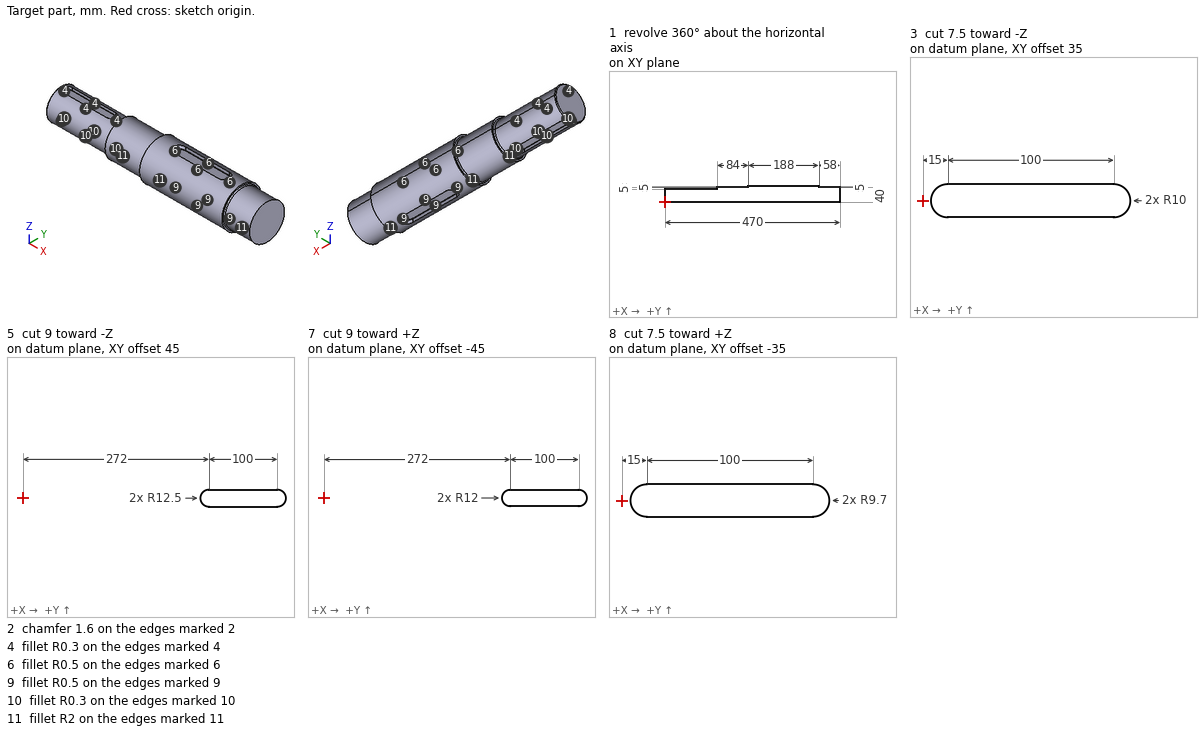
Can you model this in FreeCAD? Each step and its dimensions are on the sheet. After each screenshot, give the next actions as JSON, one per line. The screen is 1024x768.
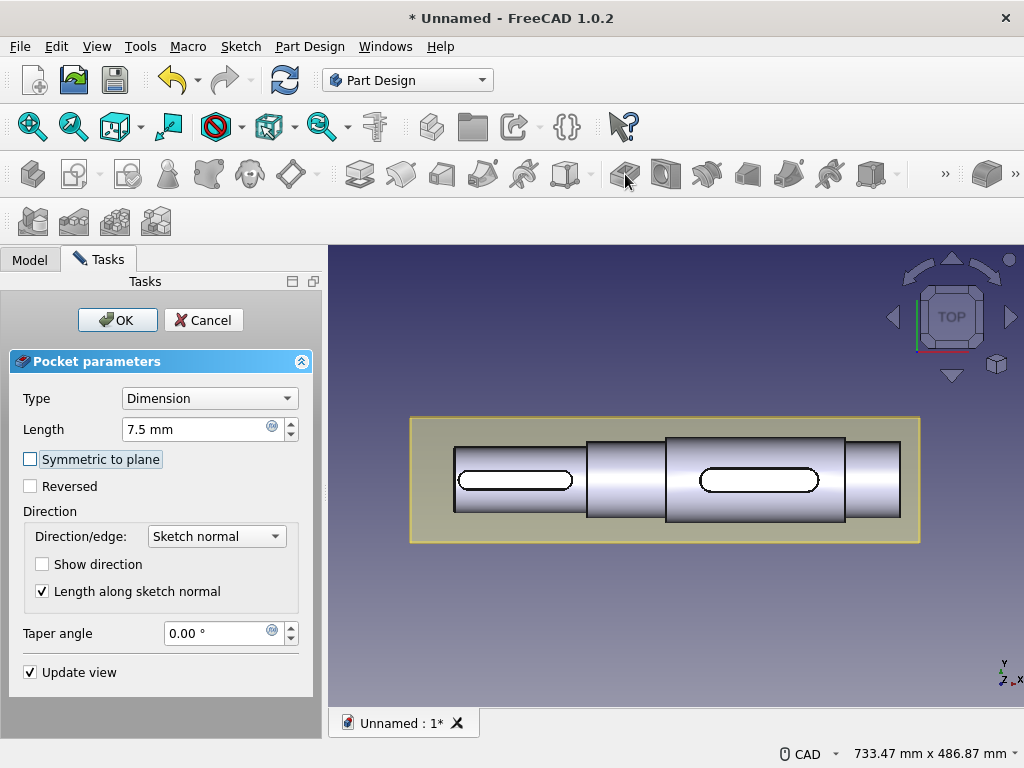
{"action": "left_click", "coordinate": [31, 486]}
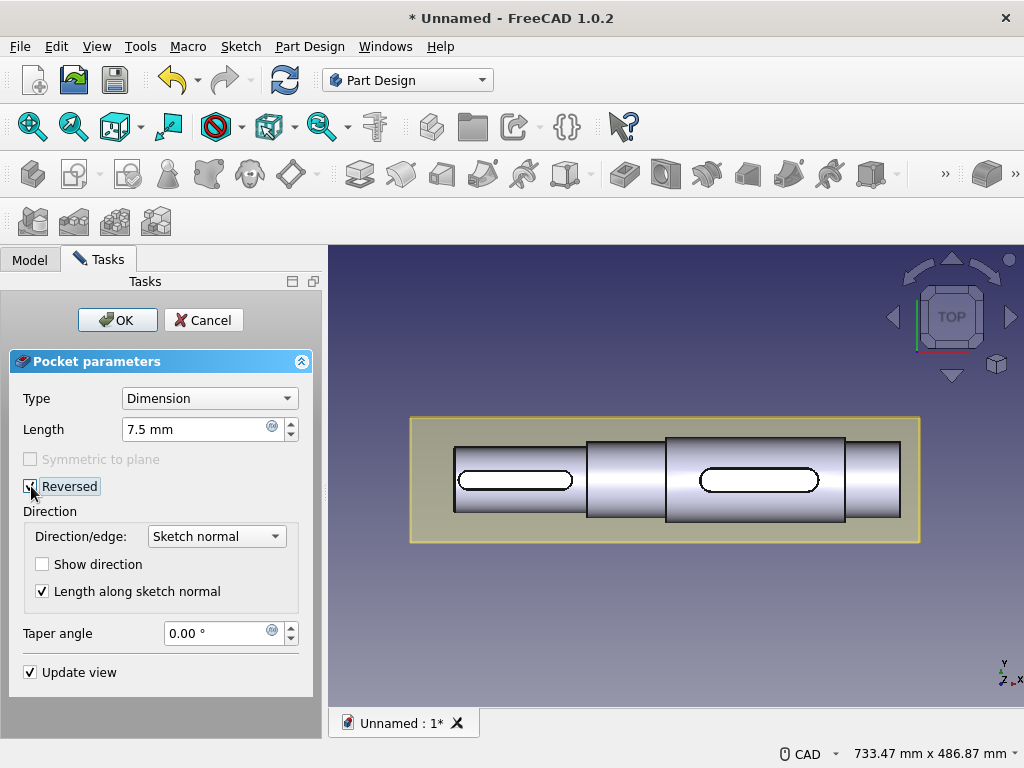
{"action": "left_click", "coordinate": [118, 320]}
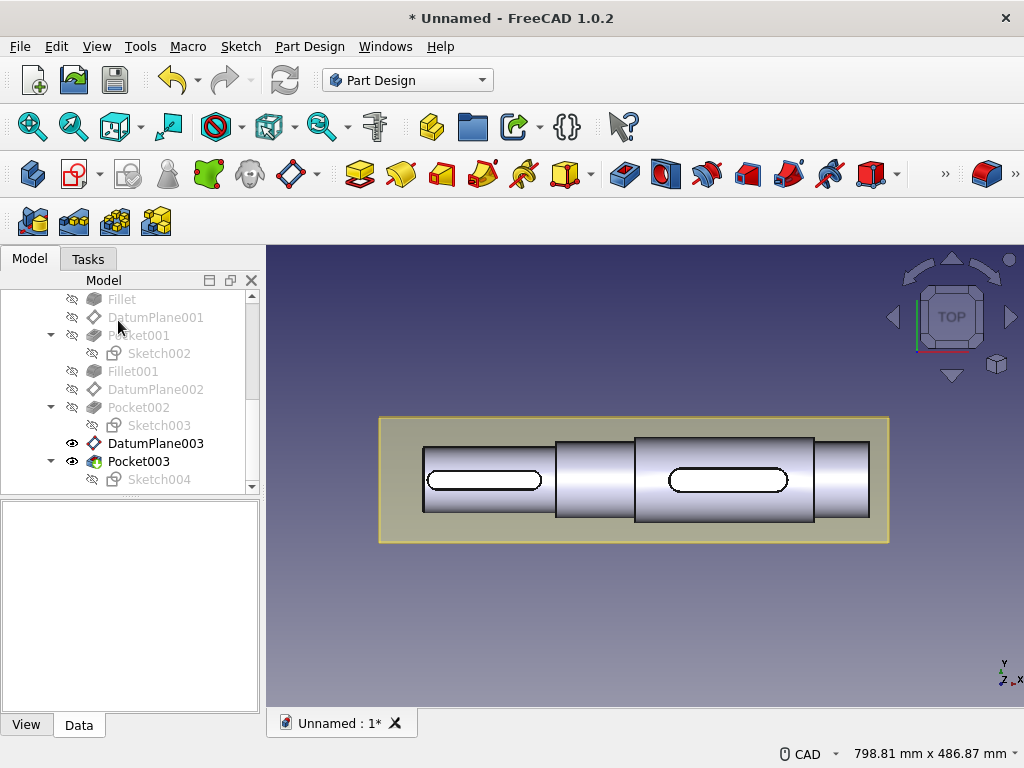
{"action": "left_click", "coordinate": [117, 443]}
{"action": "key", "text": "space"}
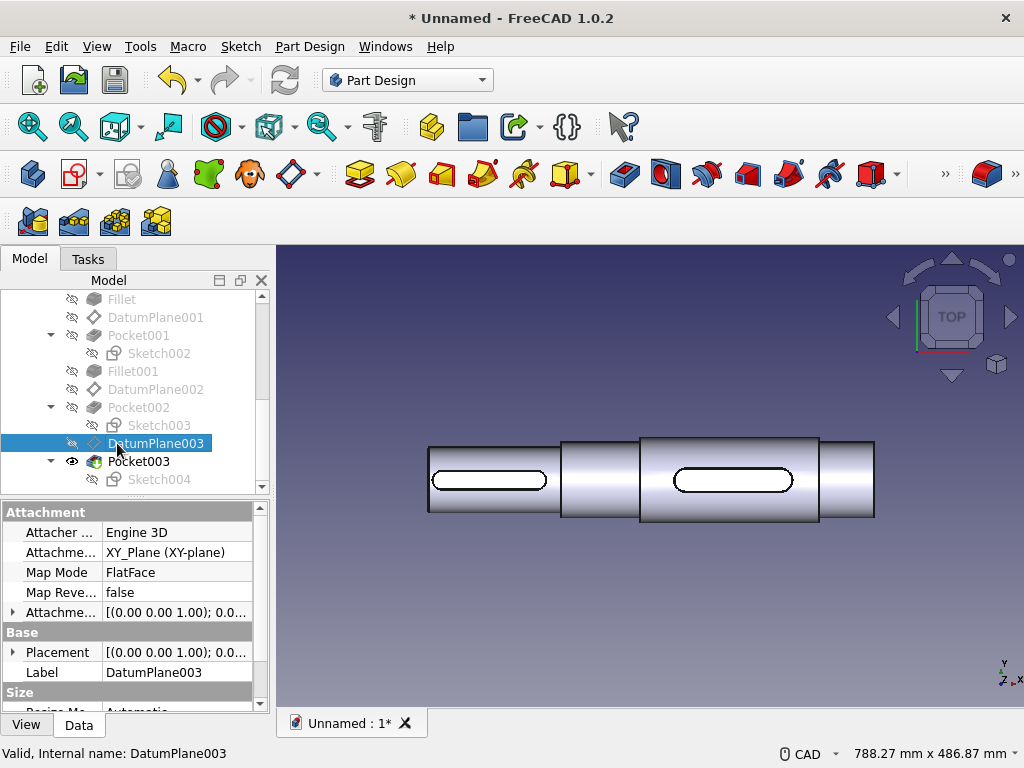
{"action": "key", "text": "0"}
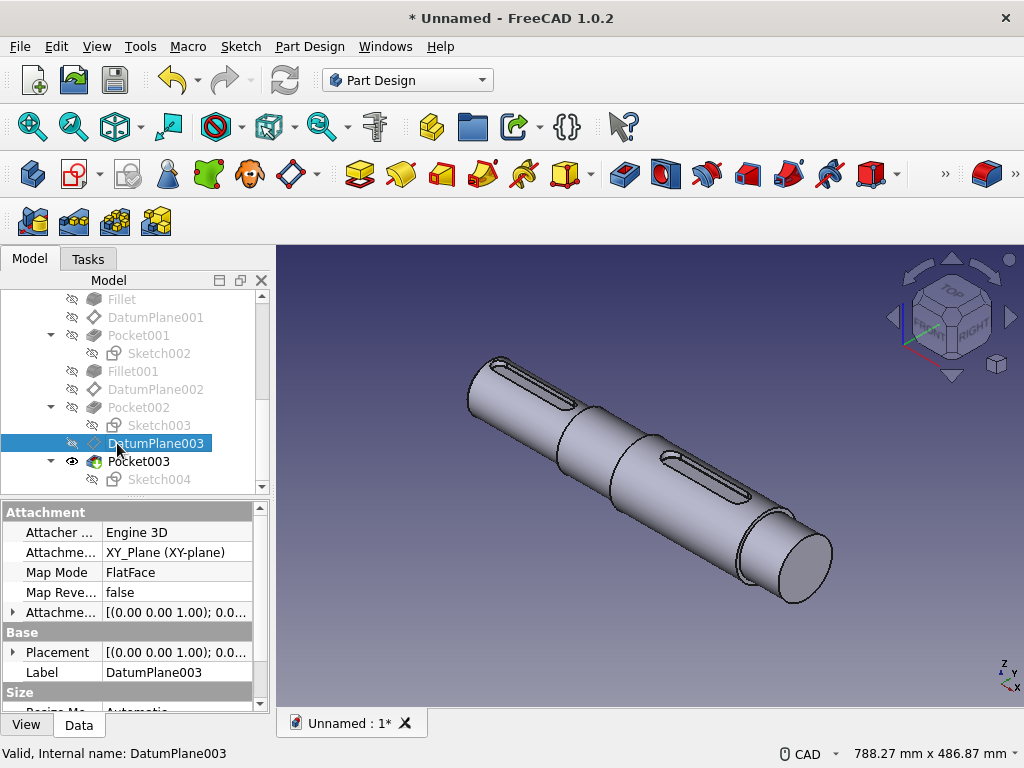
{"action": "key", "text": "2"}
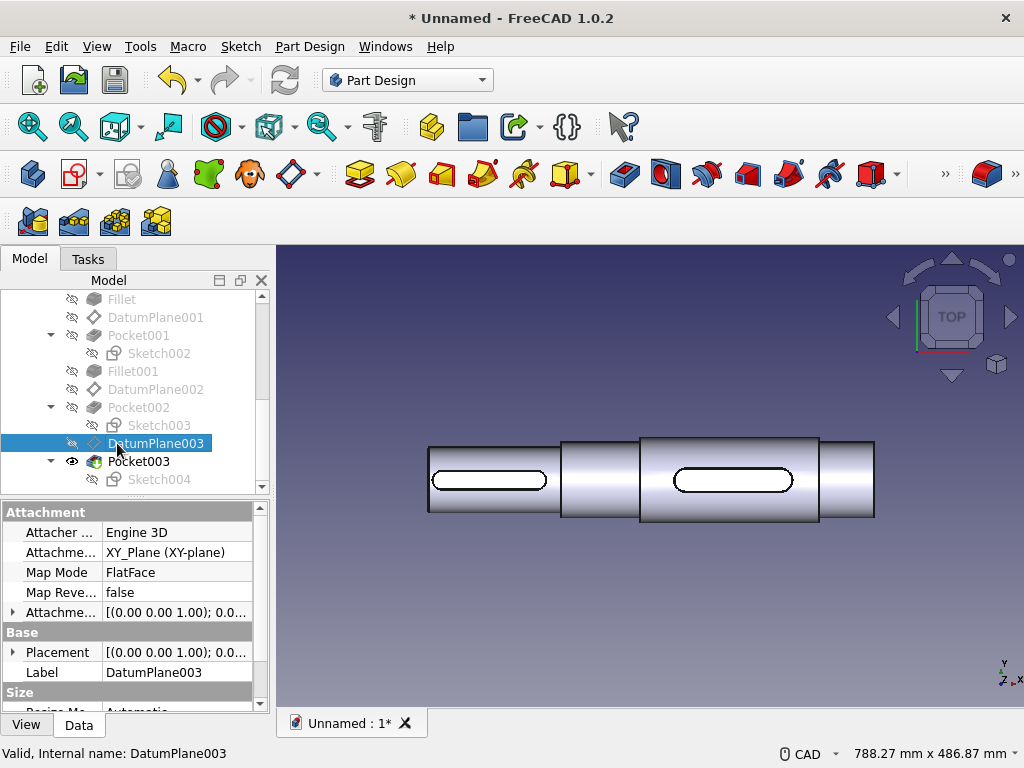
{"action": "key", "text": "1"}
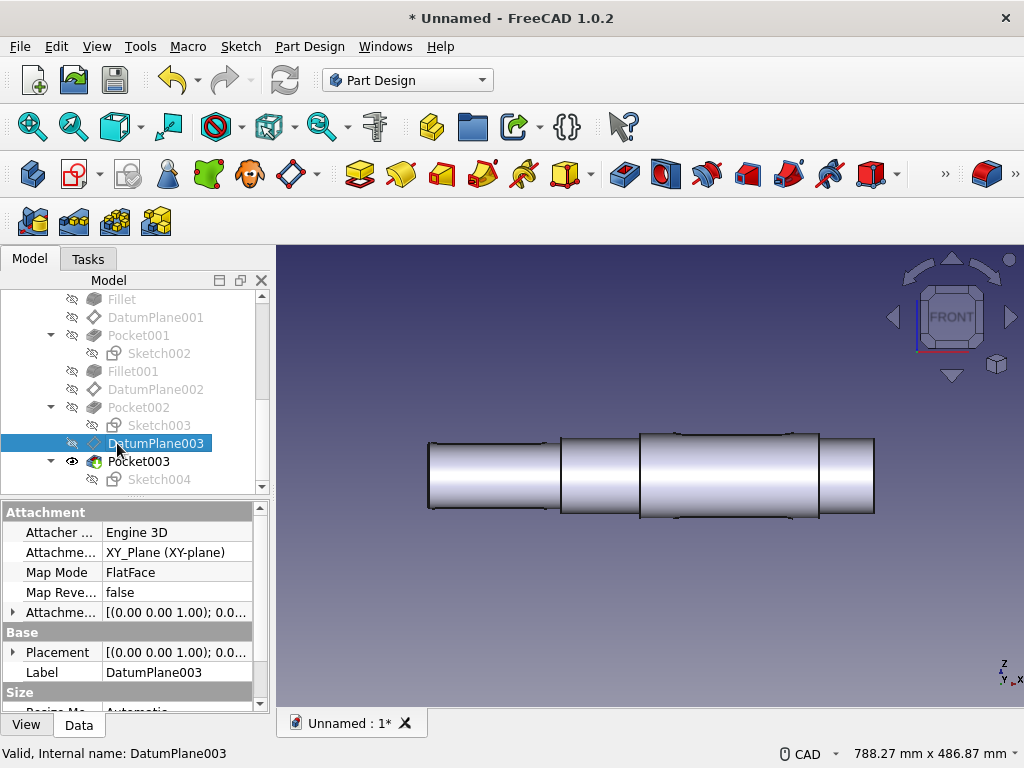
{"action": "key", "text": "3"}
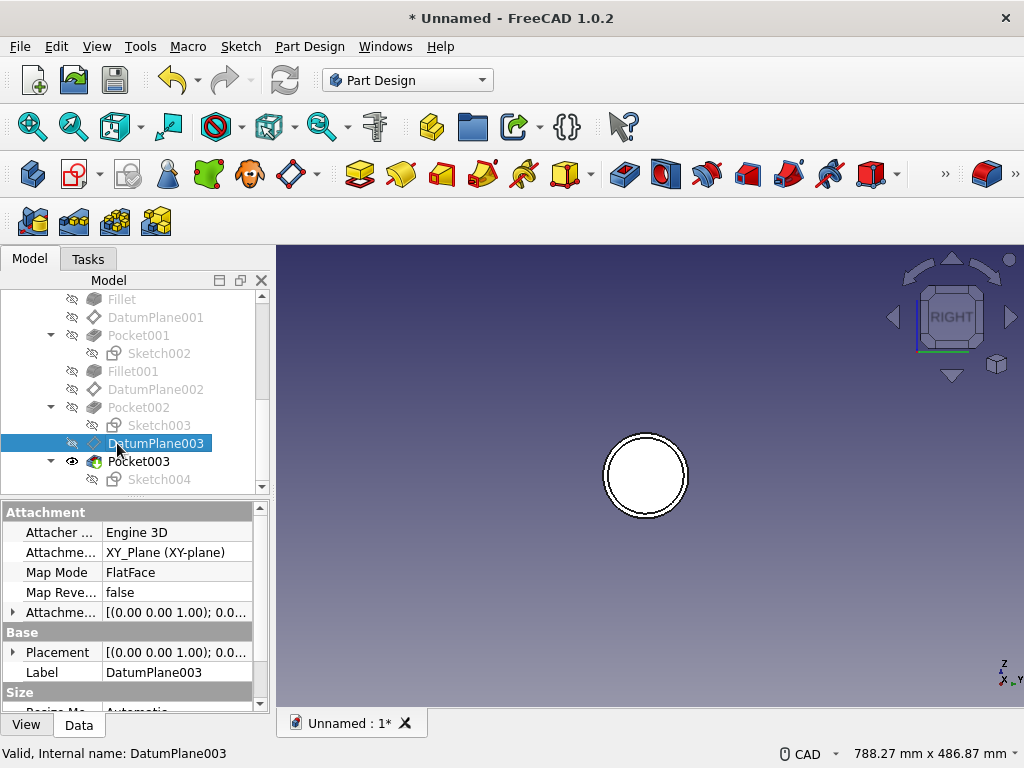
{"action": "left_click", "coordinate": [33, 128]}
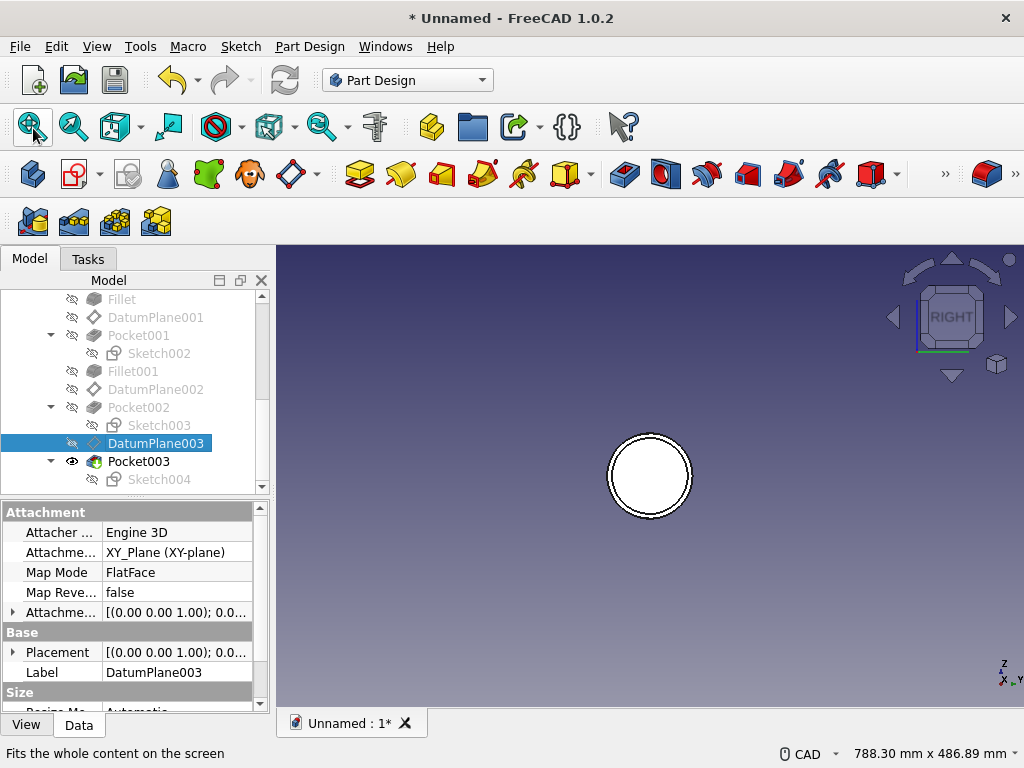
{"action": "key", "text": "5"}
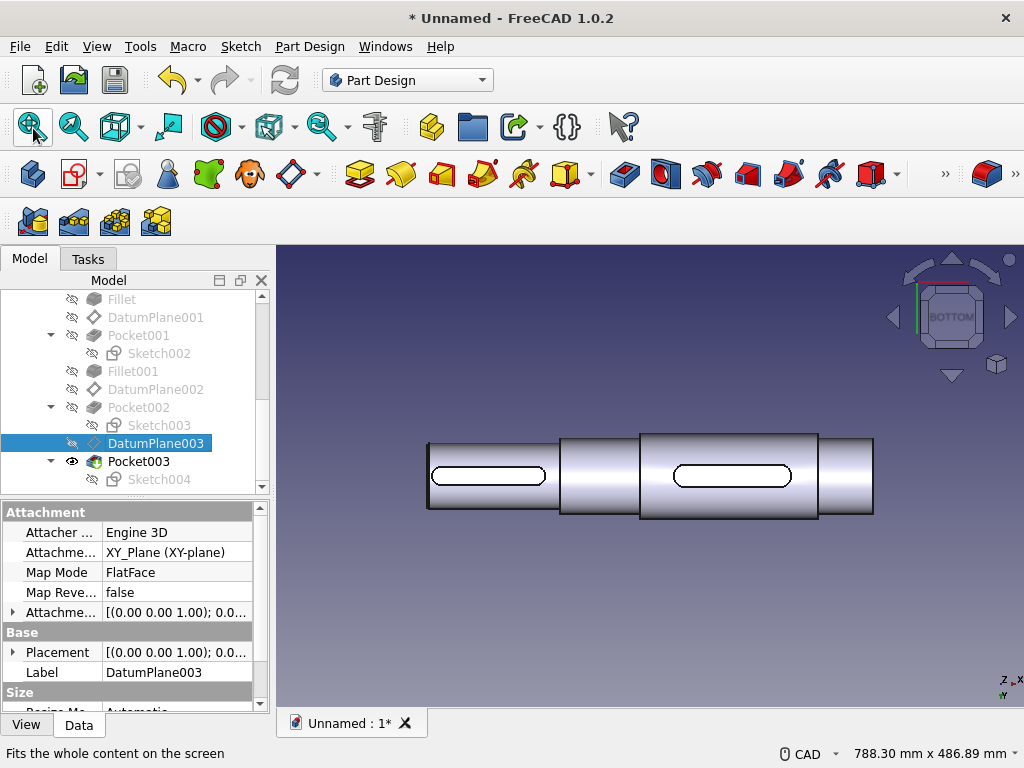
{"action": "left_click", "coordinate": [766, 475]}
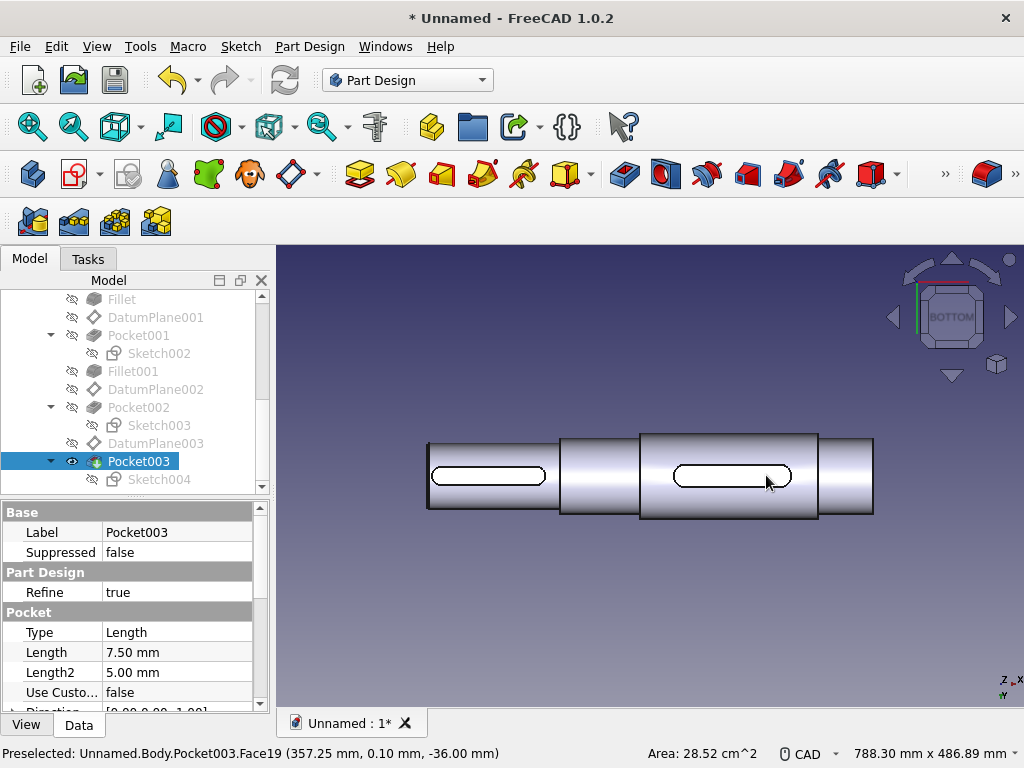
{"action": "left_click", "coordinate": [987, 174]}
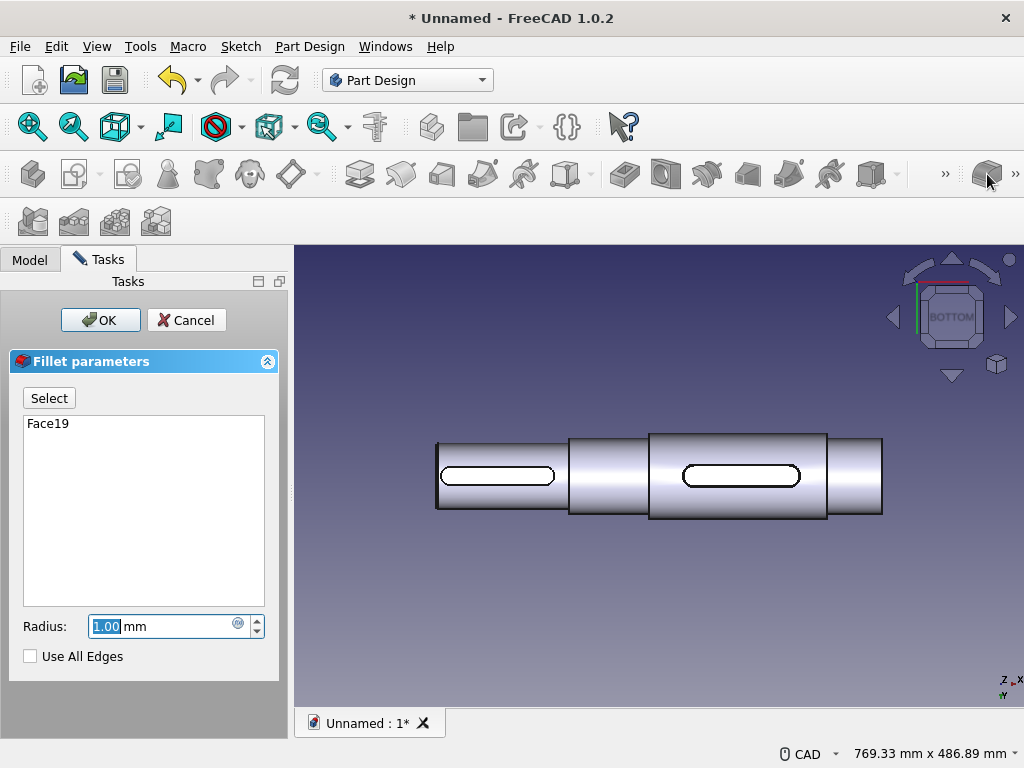
{"action": "type", "text": "0.5"}
{"action": "key", "text": "Tab"}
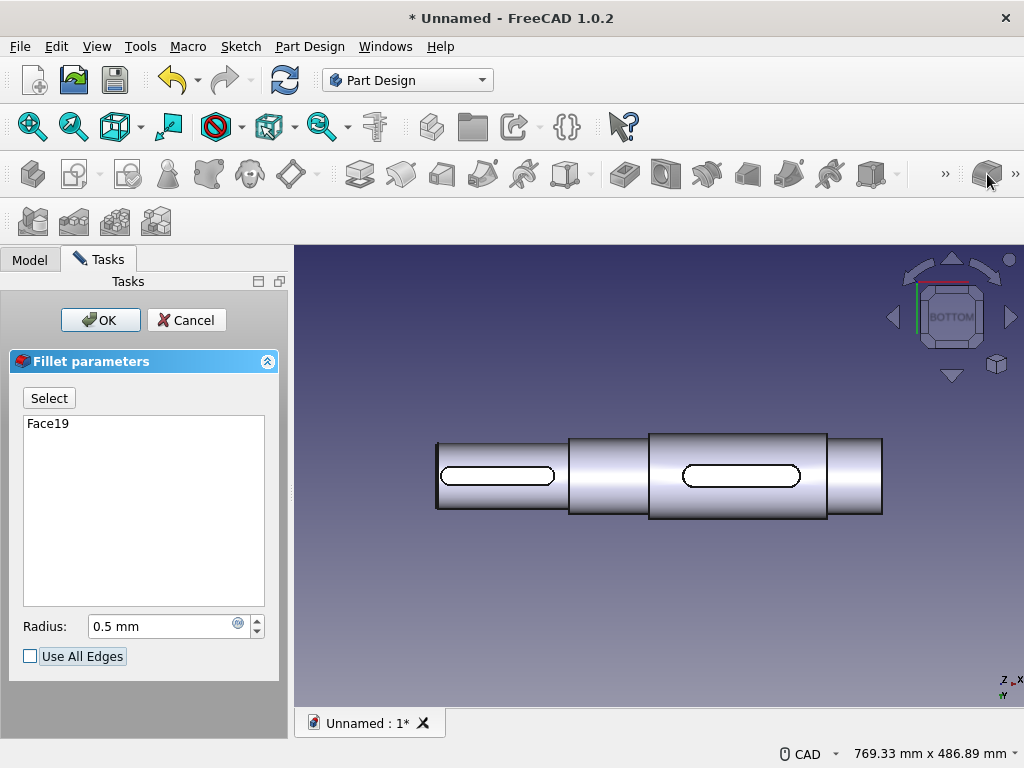
{"action": "left_click", "coordinate": [101, 320]}